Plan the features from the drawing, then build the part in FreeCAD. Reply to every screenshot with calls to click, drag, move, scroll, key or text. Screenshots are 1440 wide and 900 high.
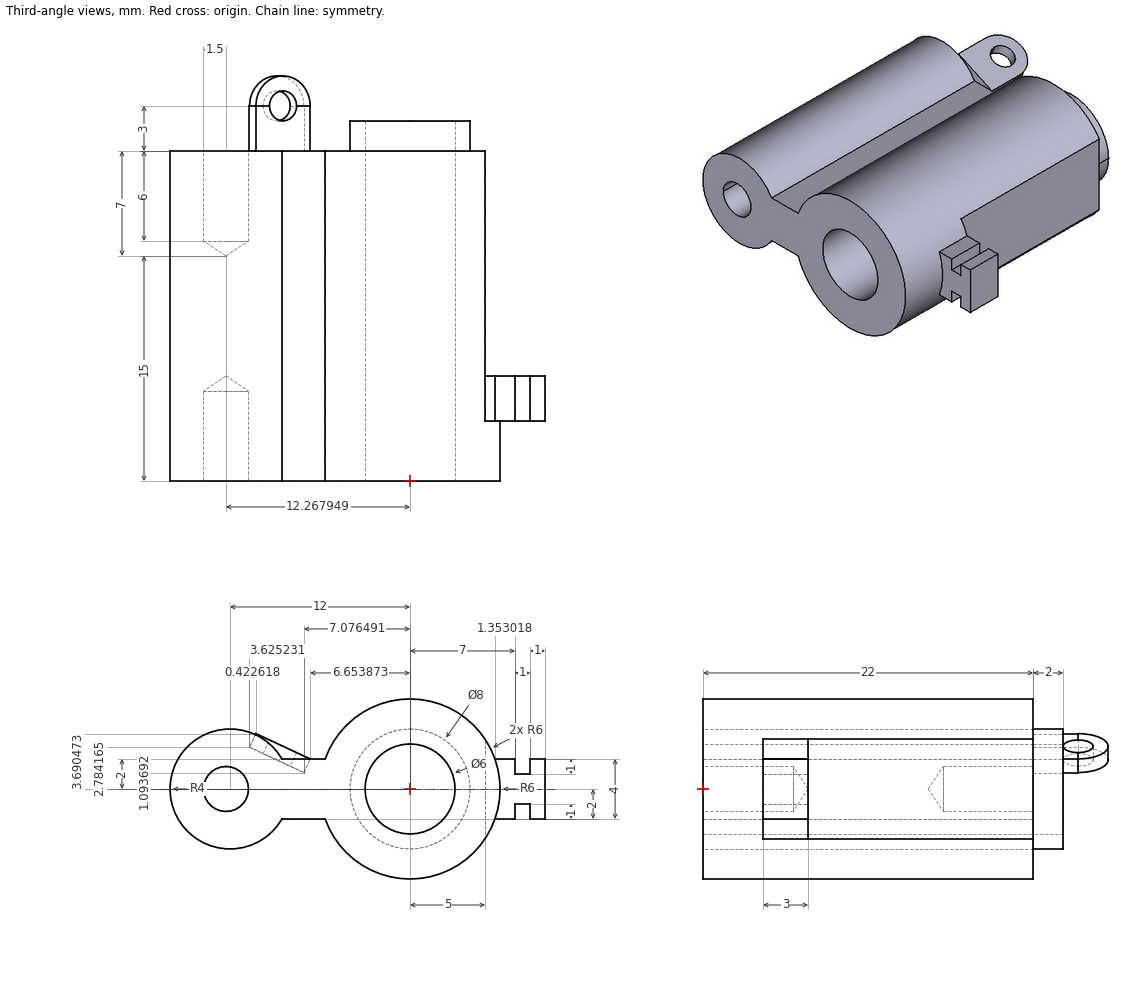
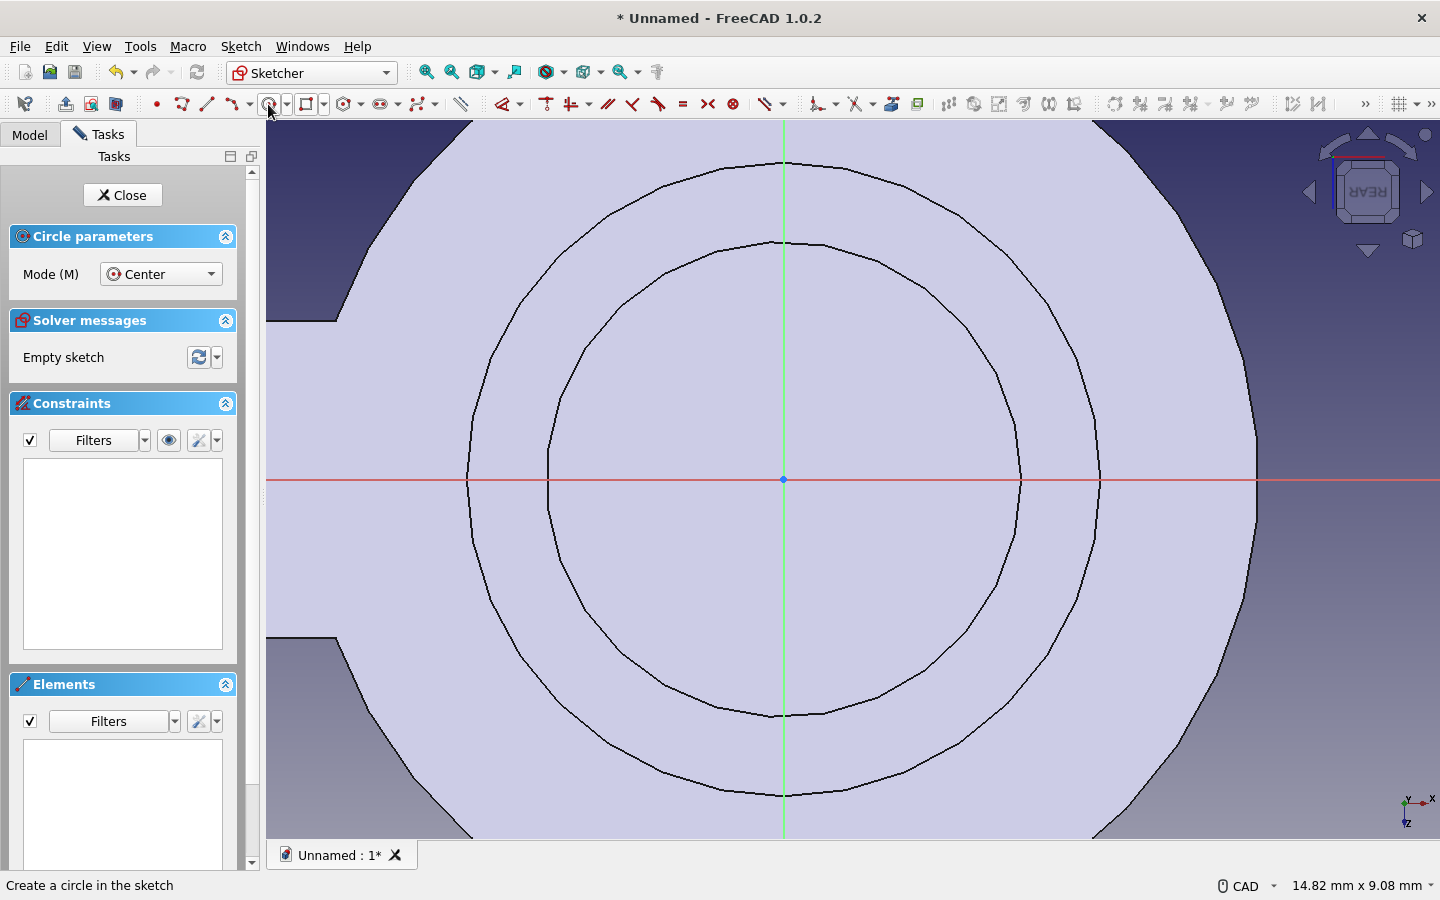
click(784, 479)
move(952, 311)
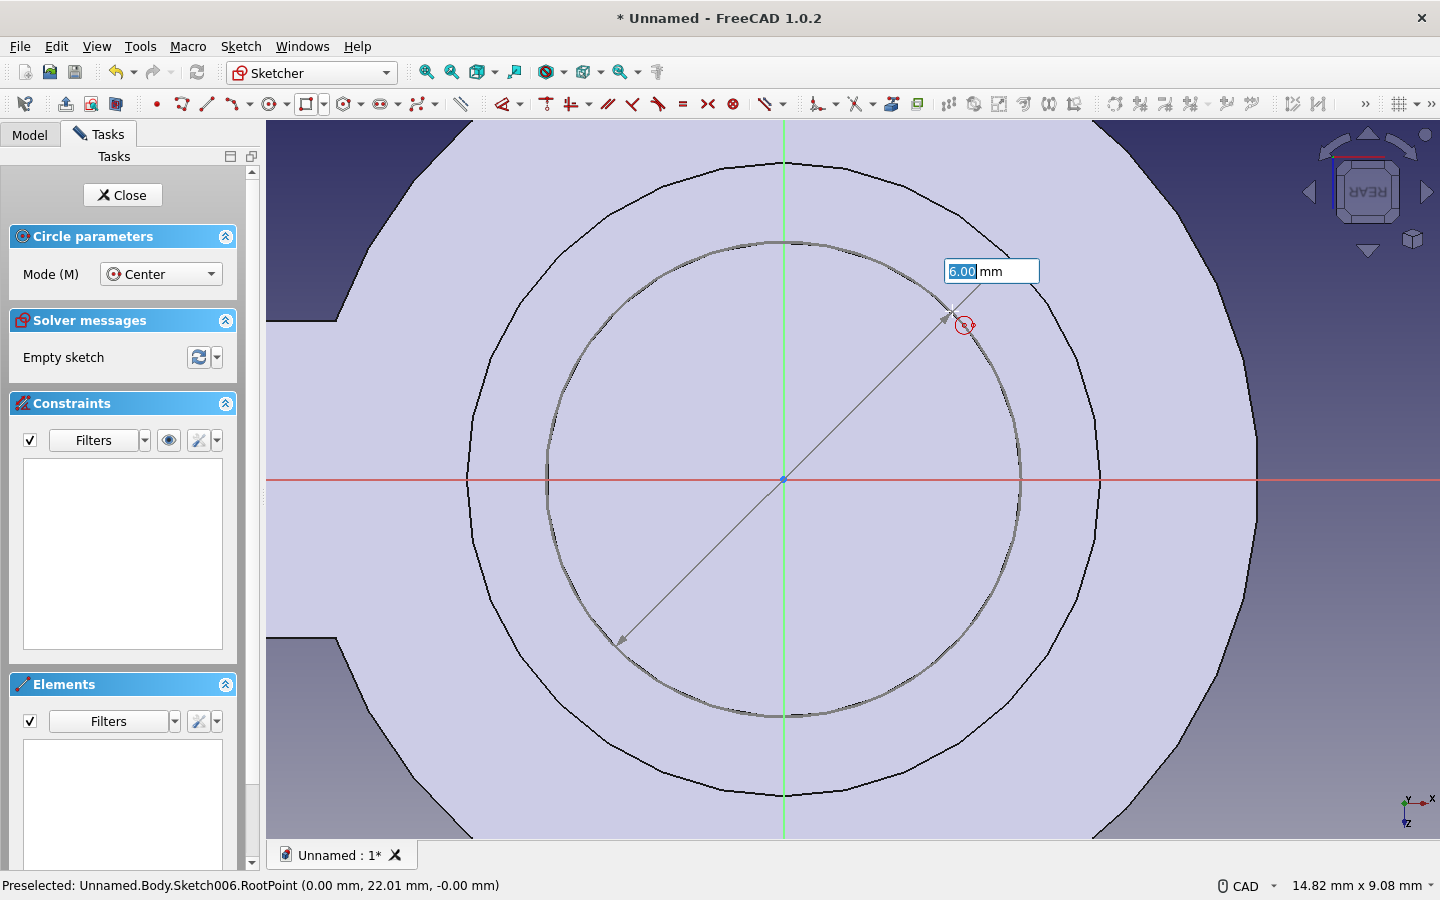
text(6)
key(Return)
key(Escape)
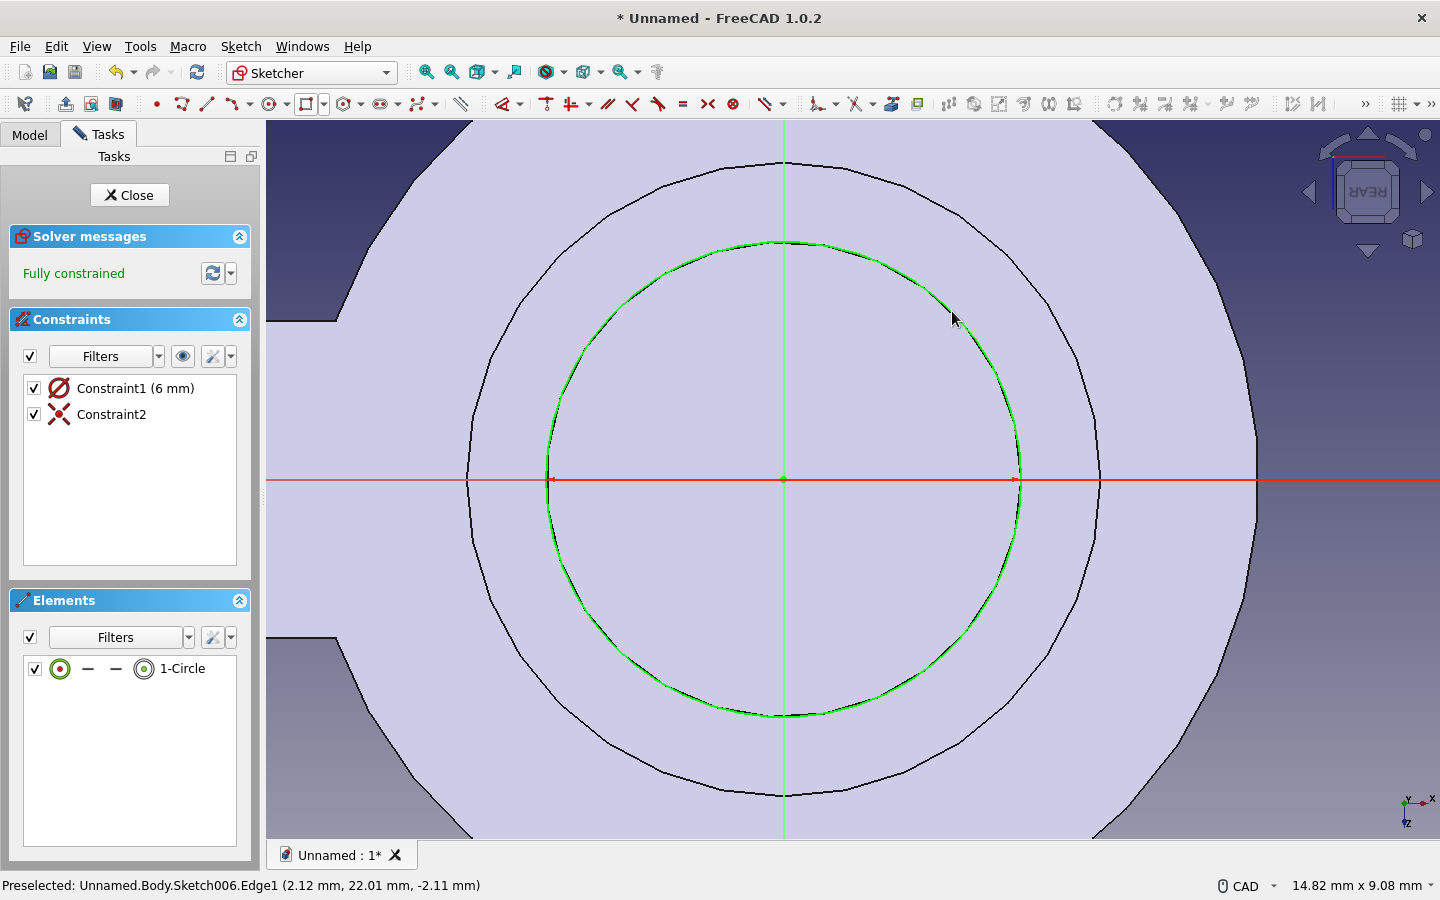
click(130, 195)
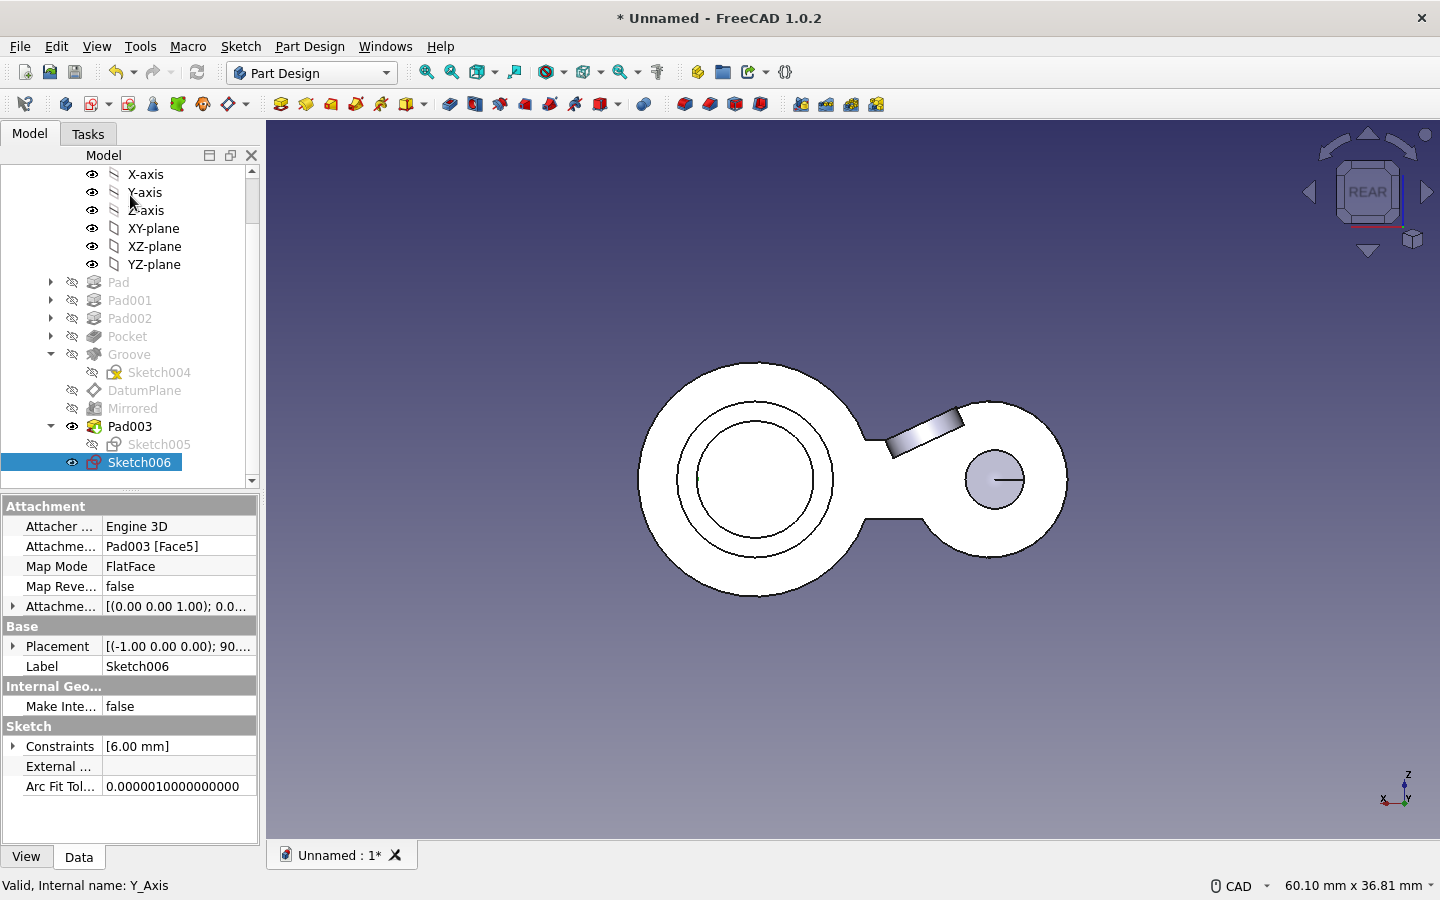
click(450, 104)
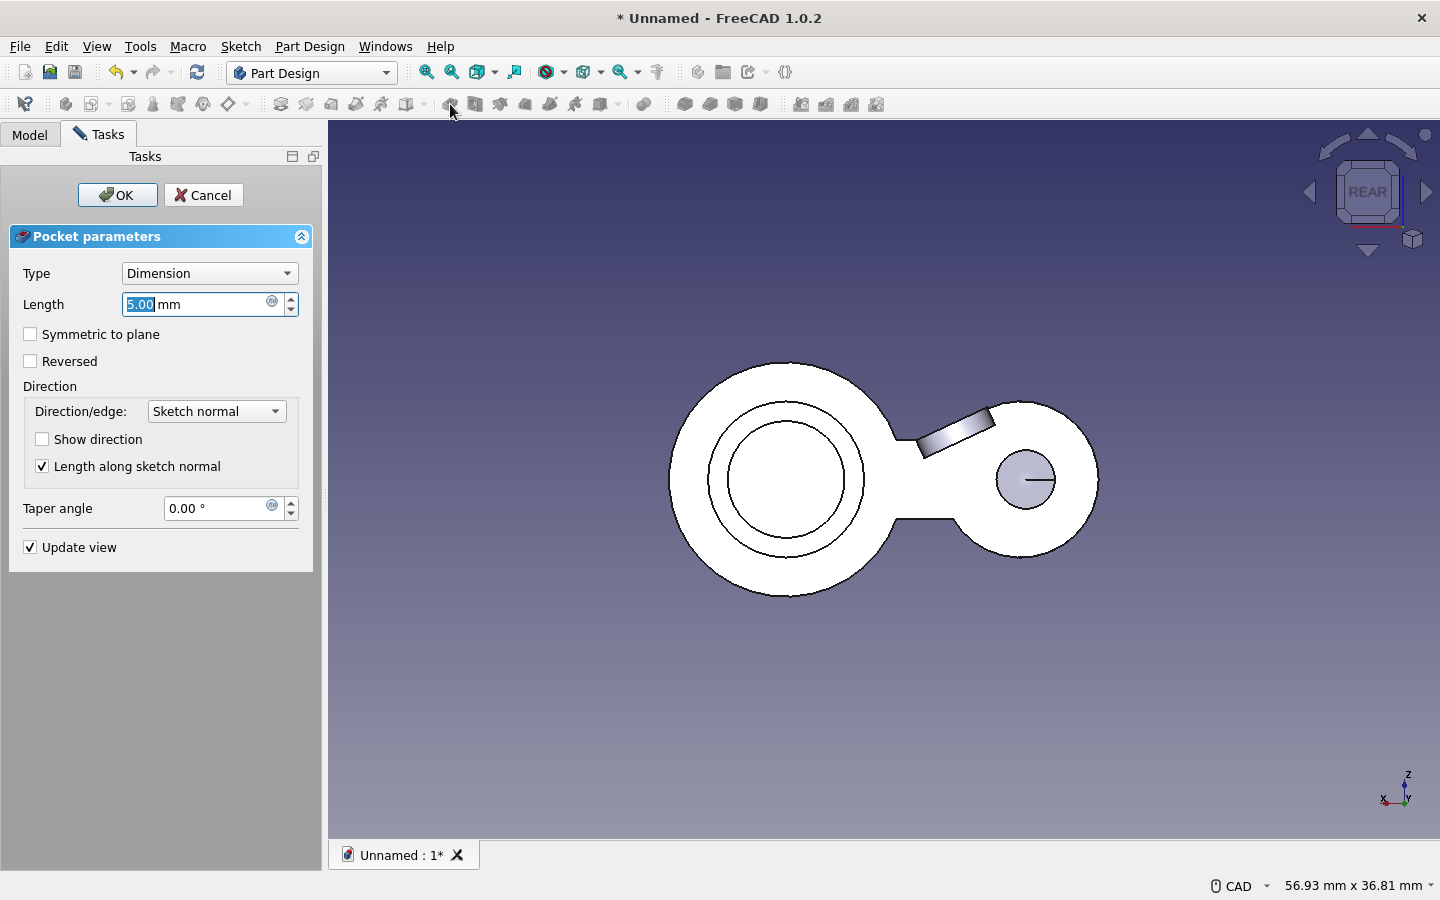
click(210, 274)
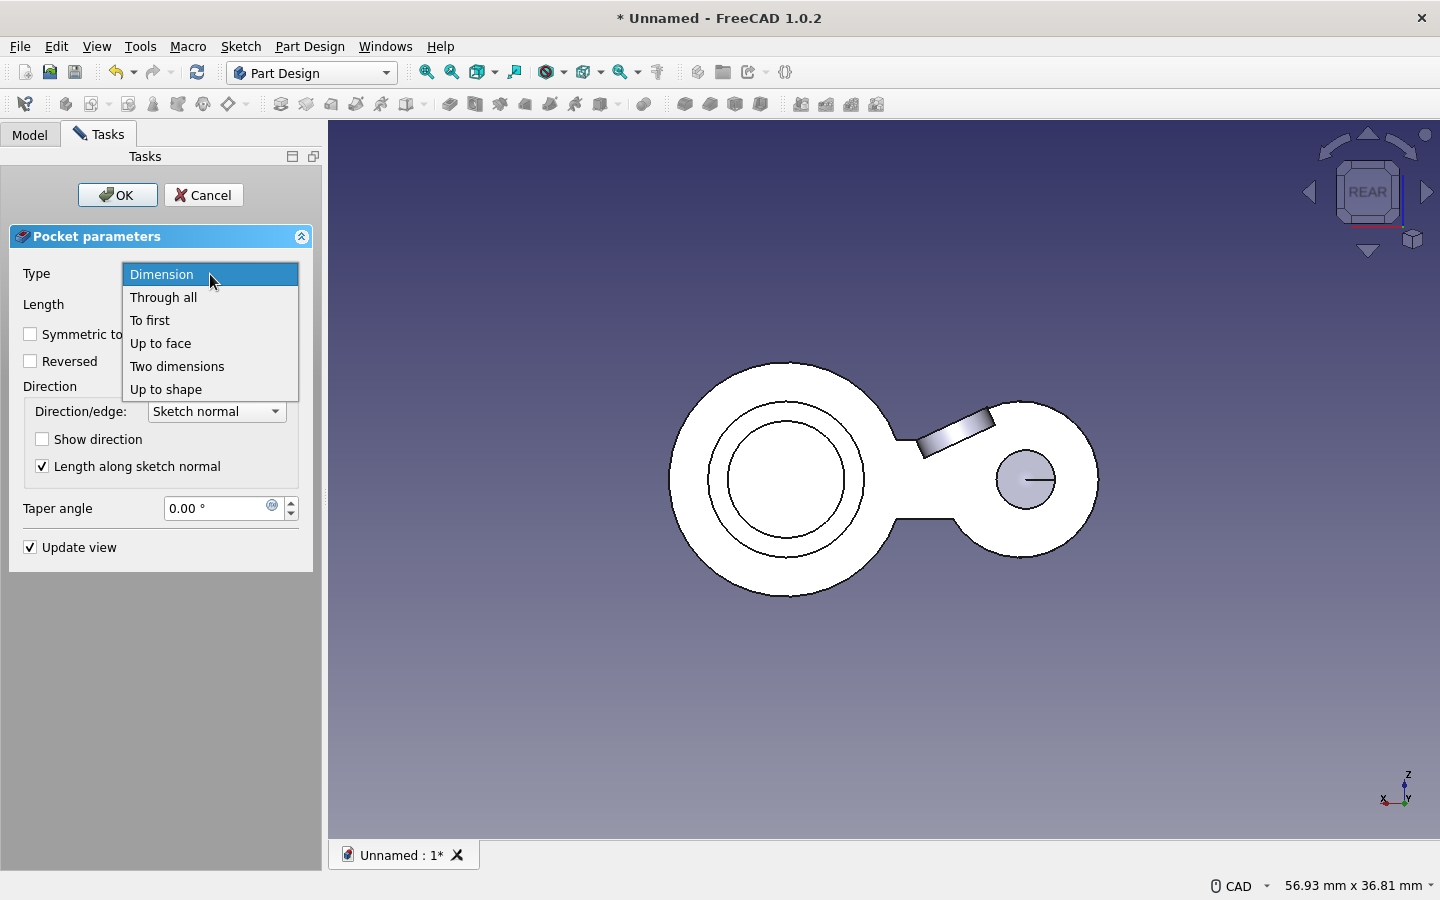
click(208, 298)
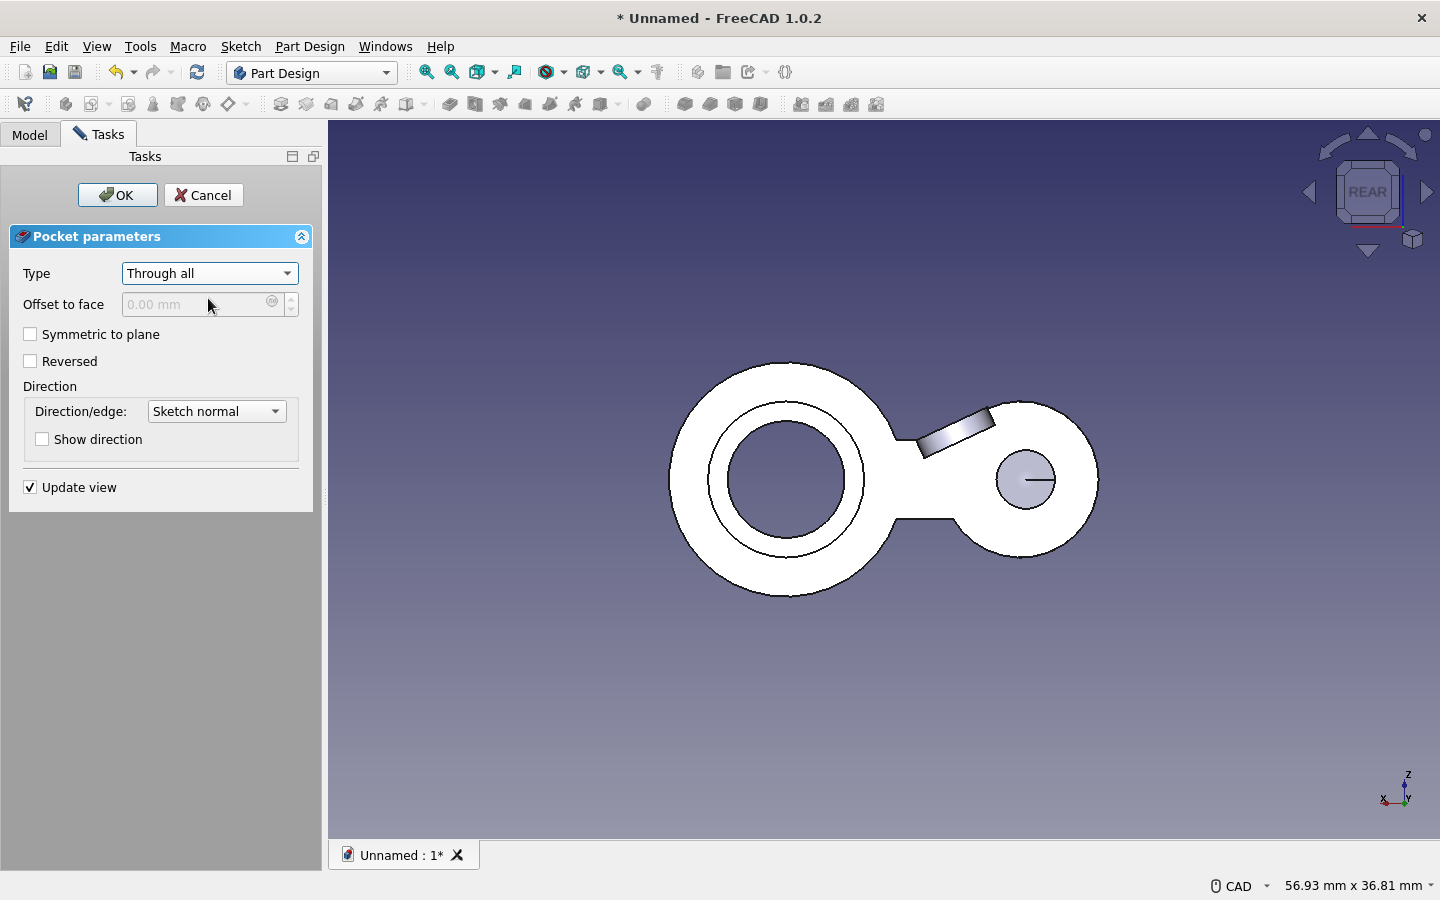
click(118, 195)